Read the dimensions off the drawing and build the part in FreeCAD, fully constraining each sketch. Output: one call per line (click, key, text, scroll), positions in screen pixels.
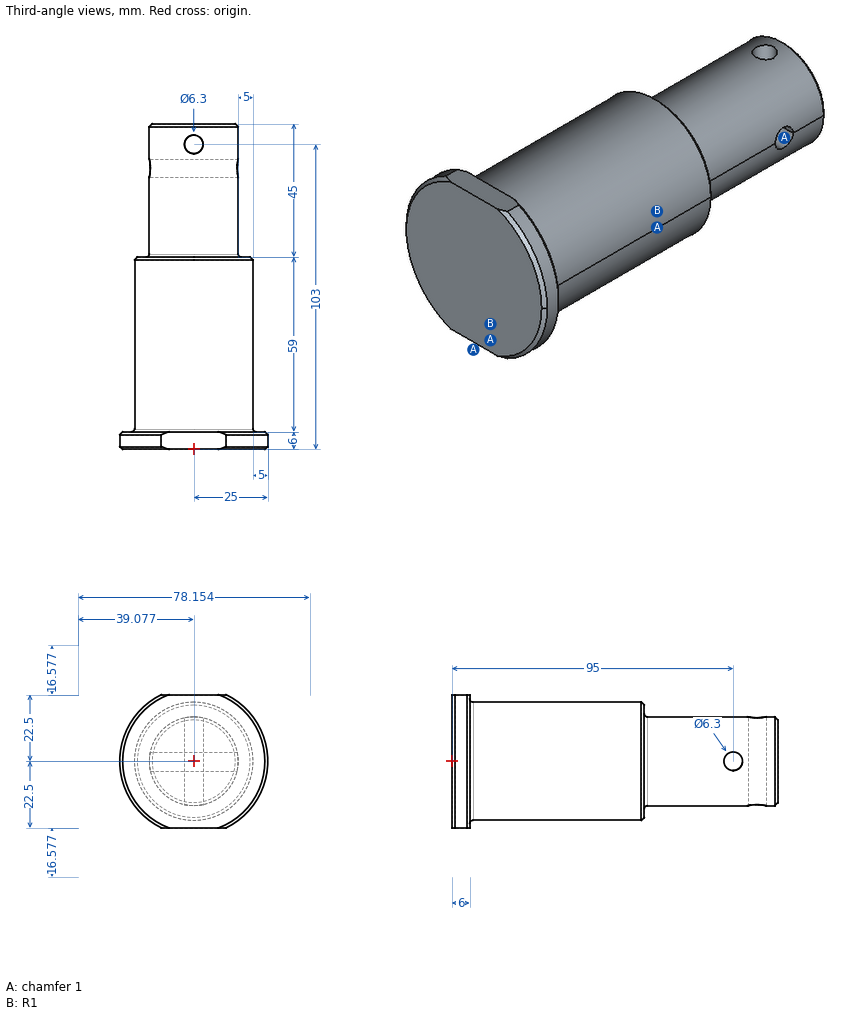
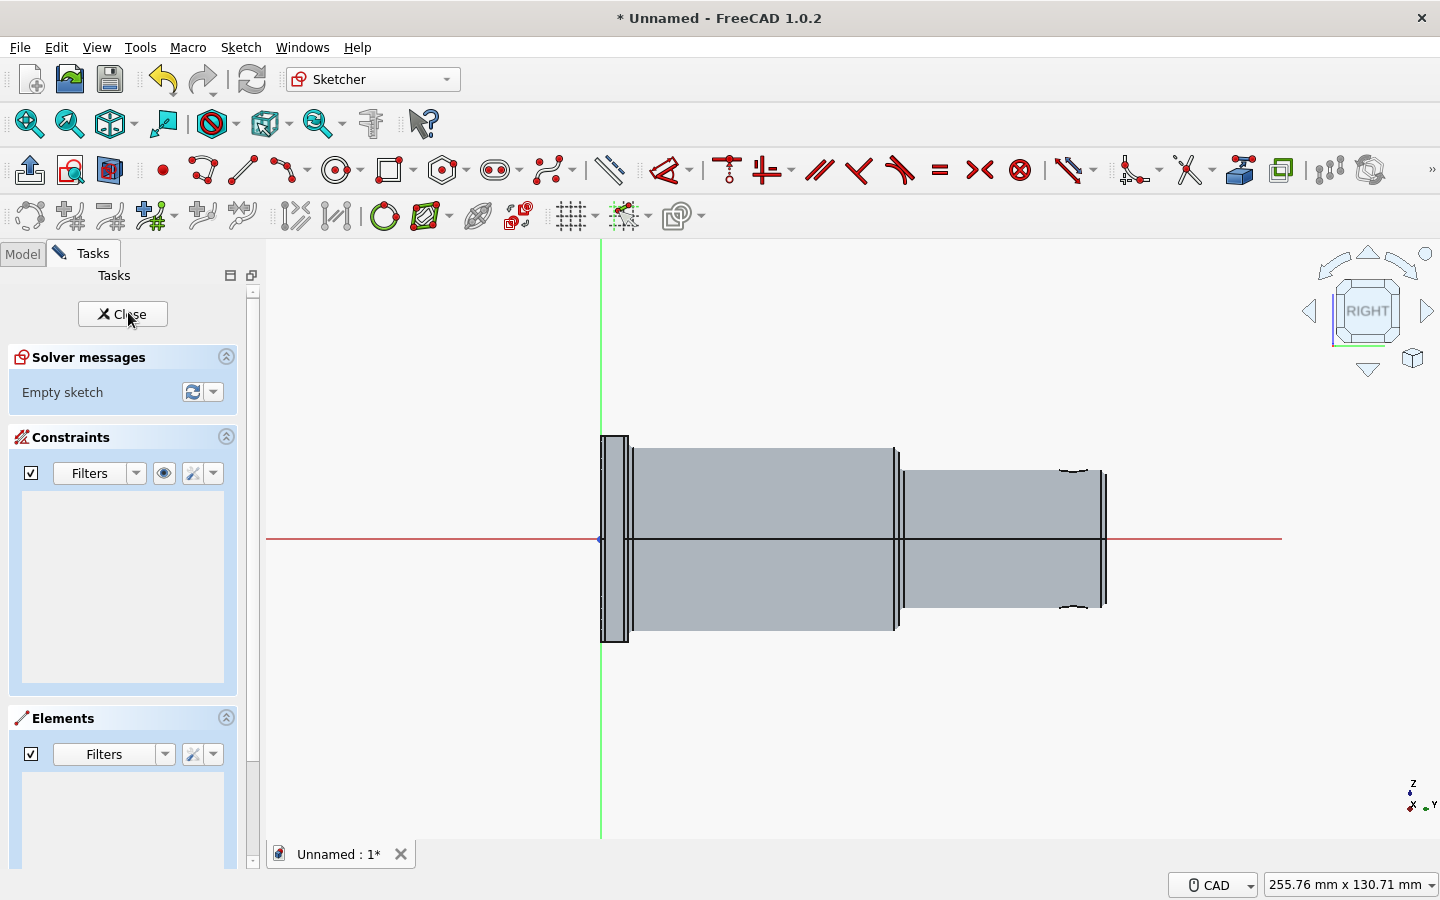
key(q)
key(s)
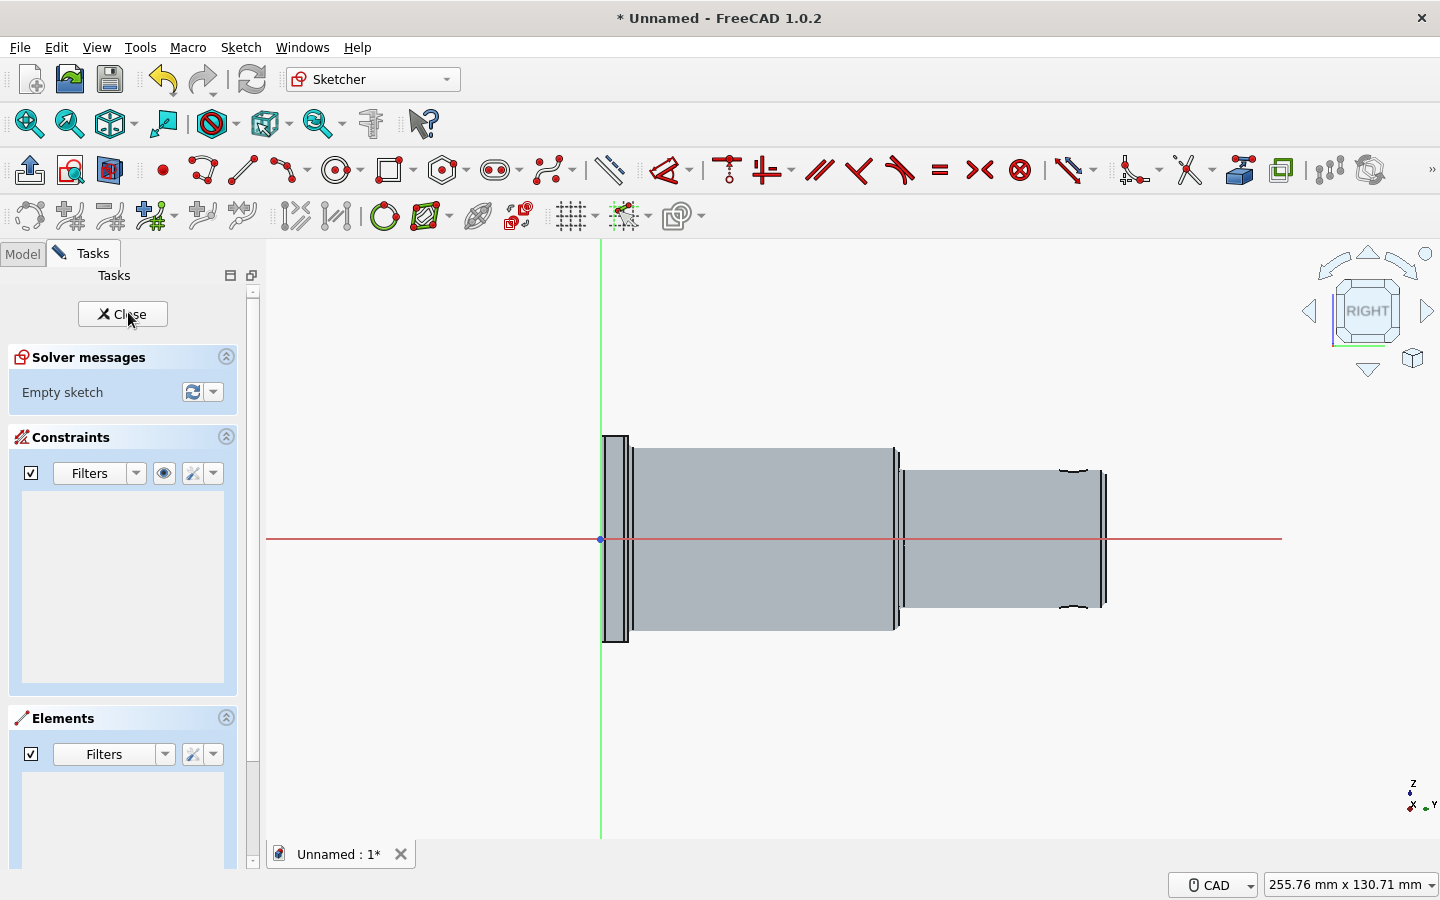
scroll(1057, 539, up, 13)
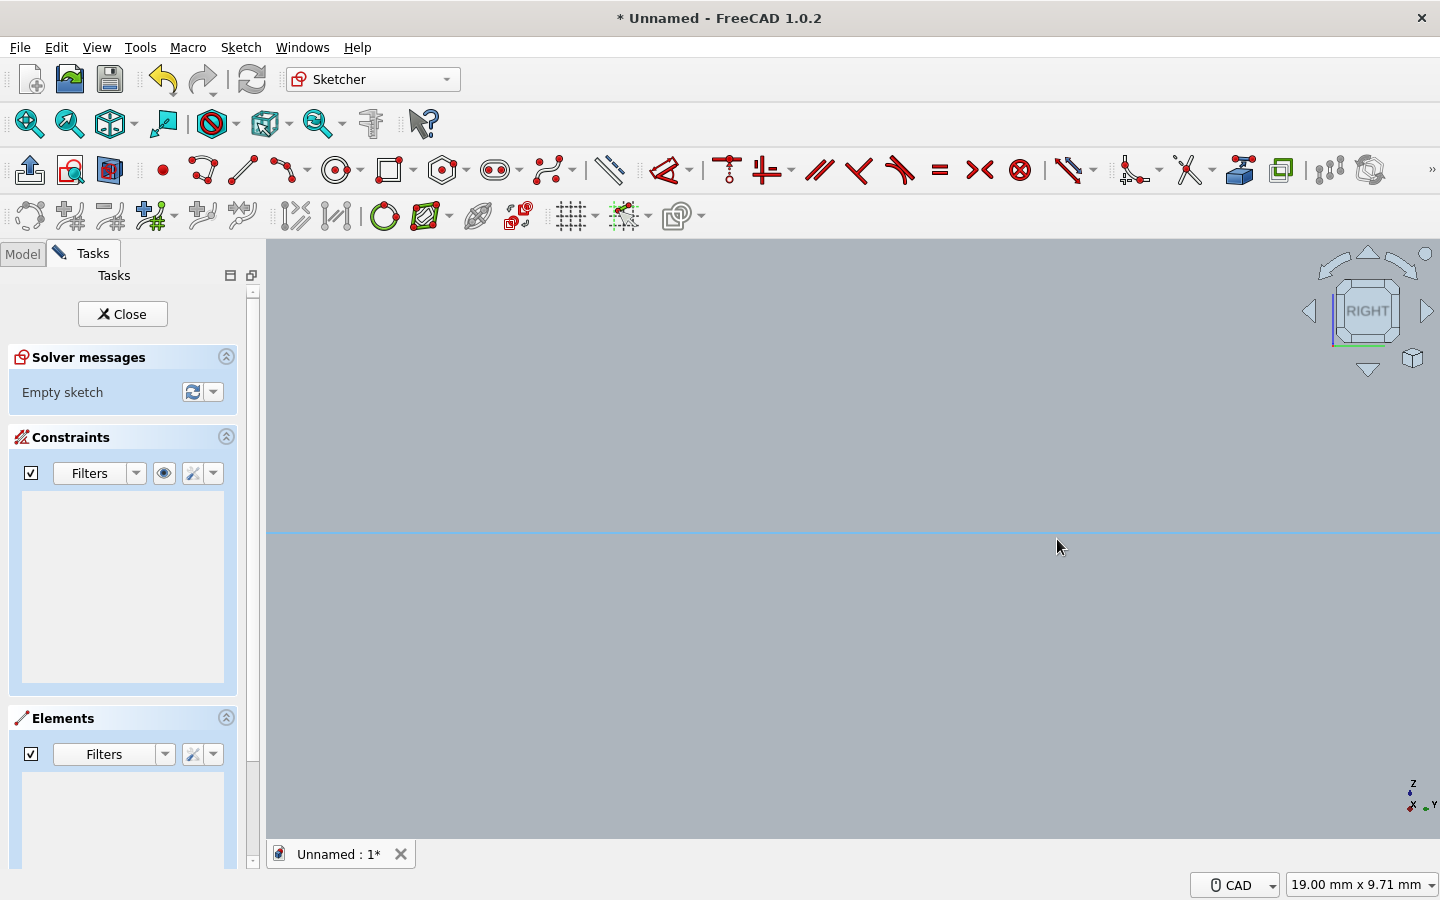
key(g)
key(c)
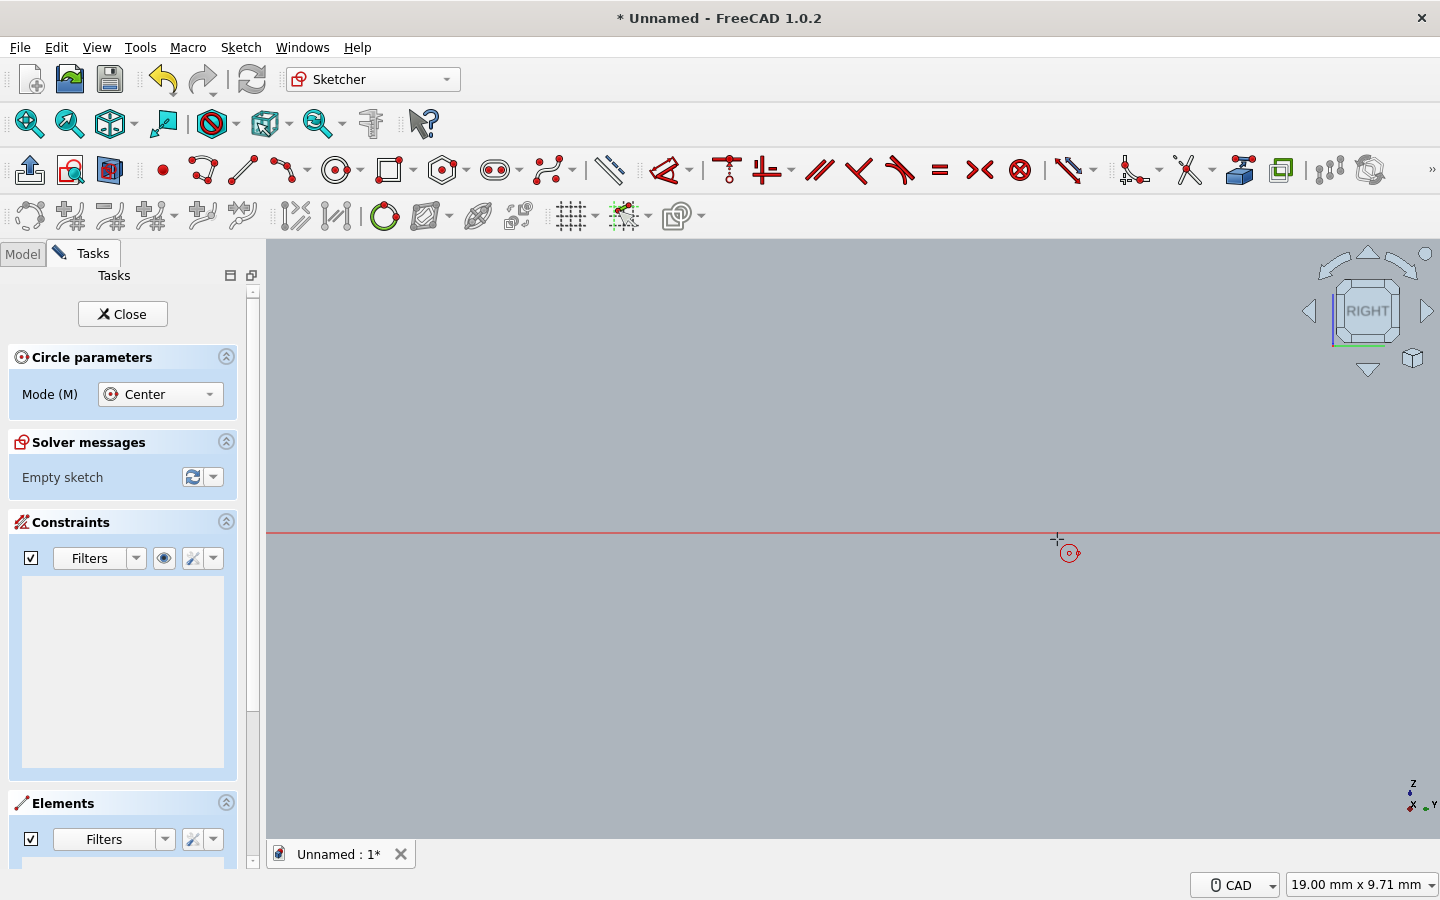
click(775, 533)
click(912, 396)
key(Escape)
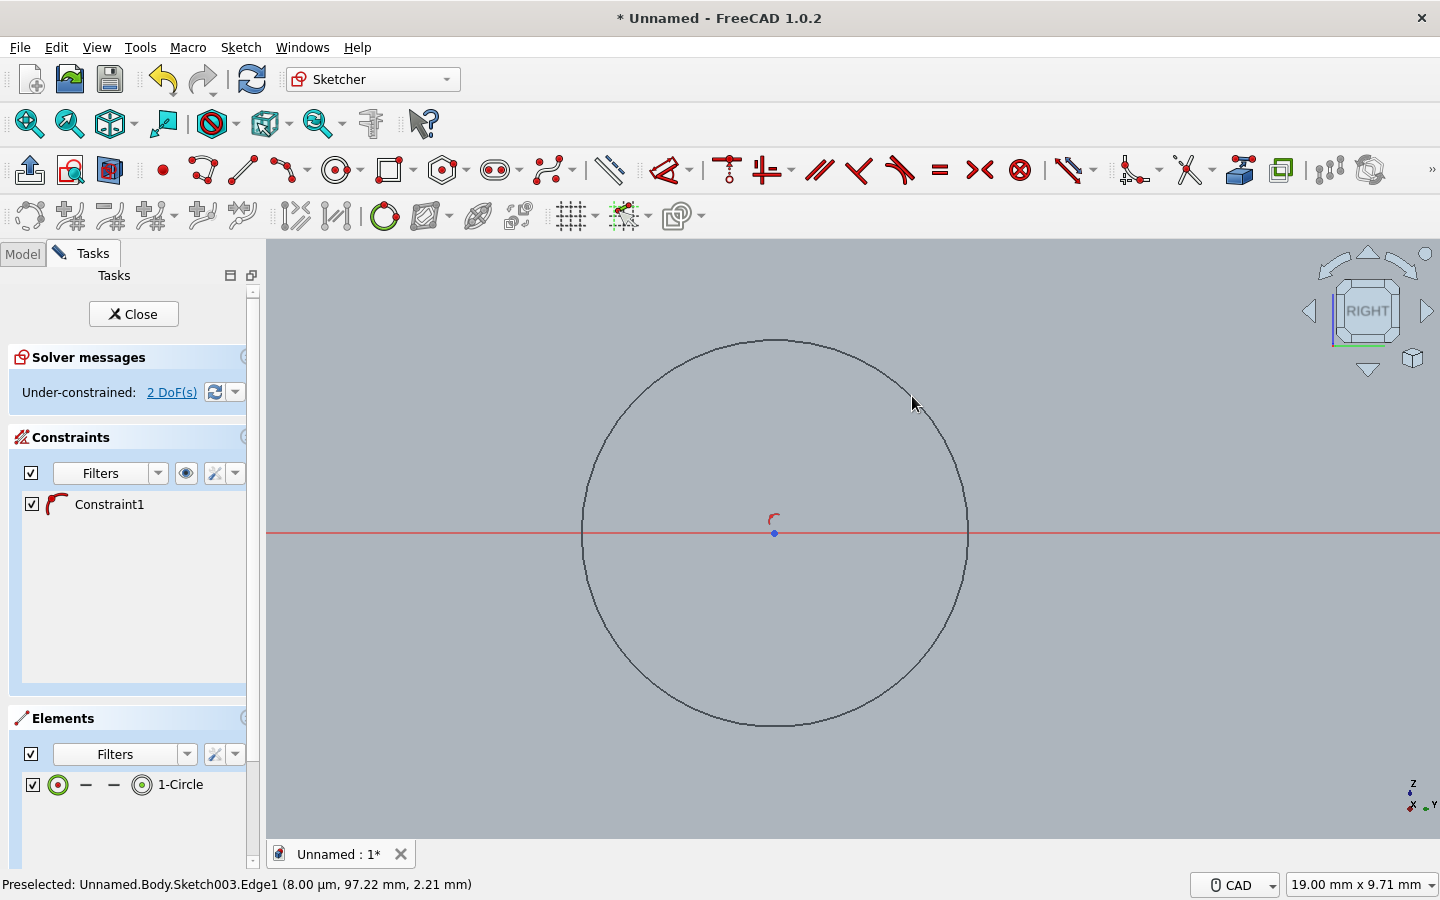
click(664, 170)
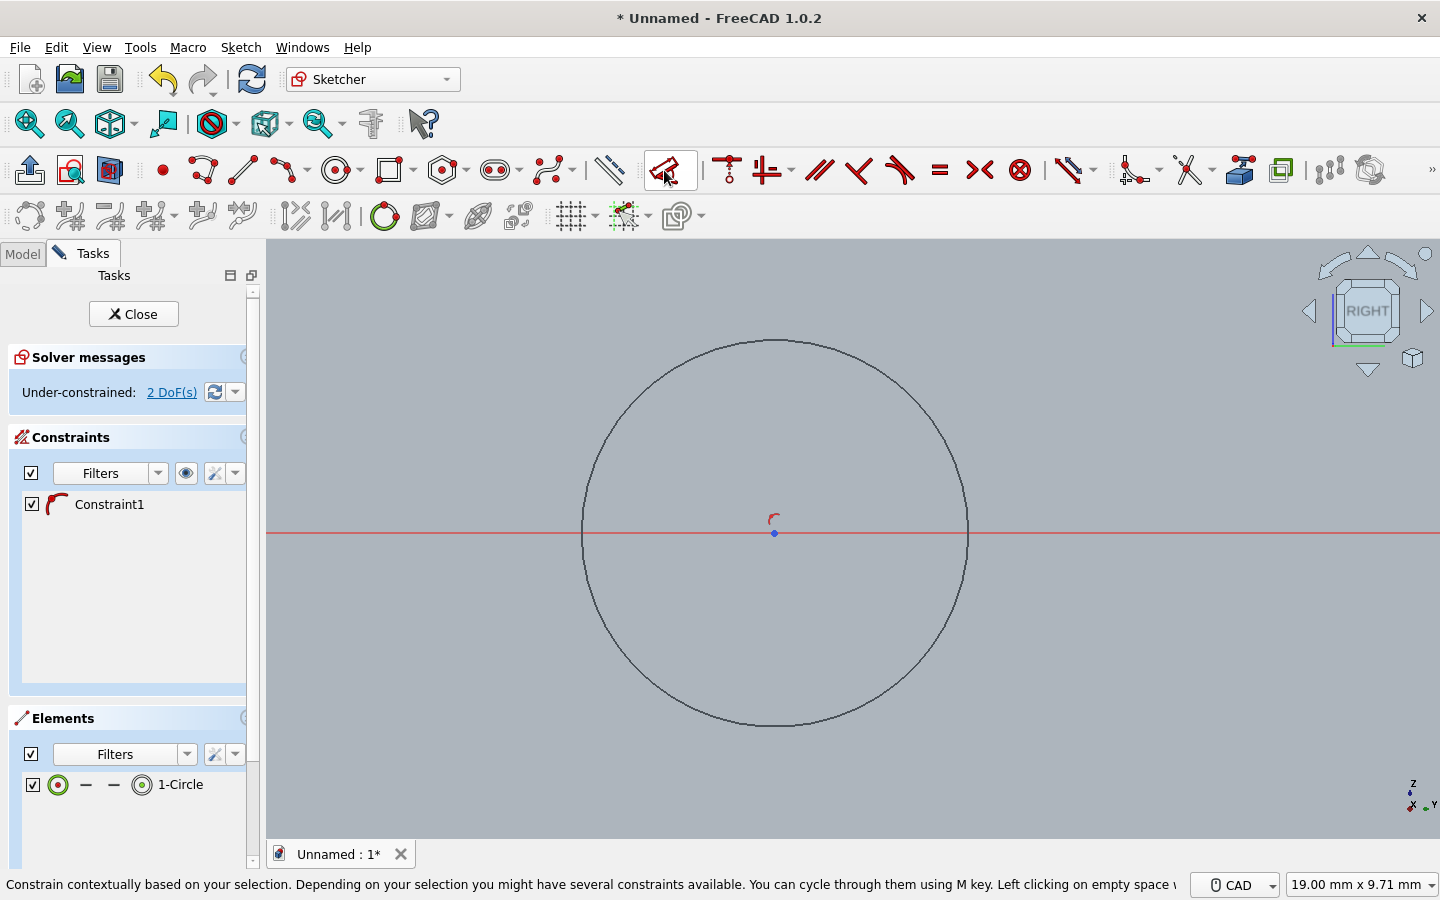
click(911, 396)
click(934, 373)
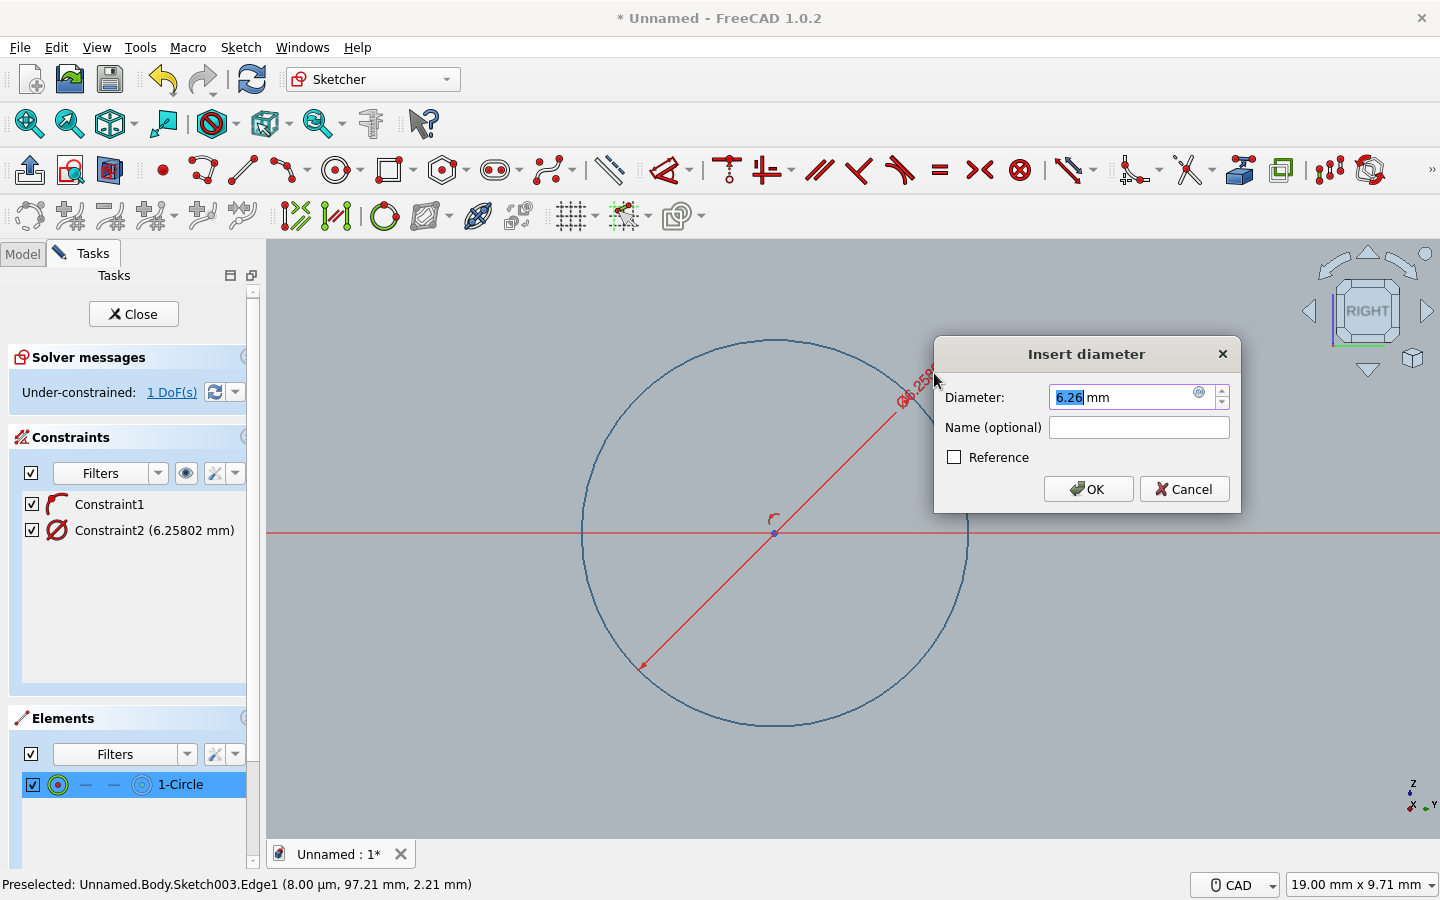
text(6.3)
key(Return)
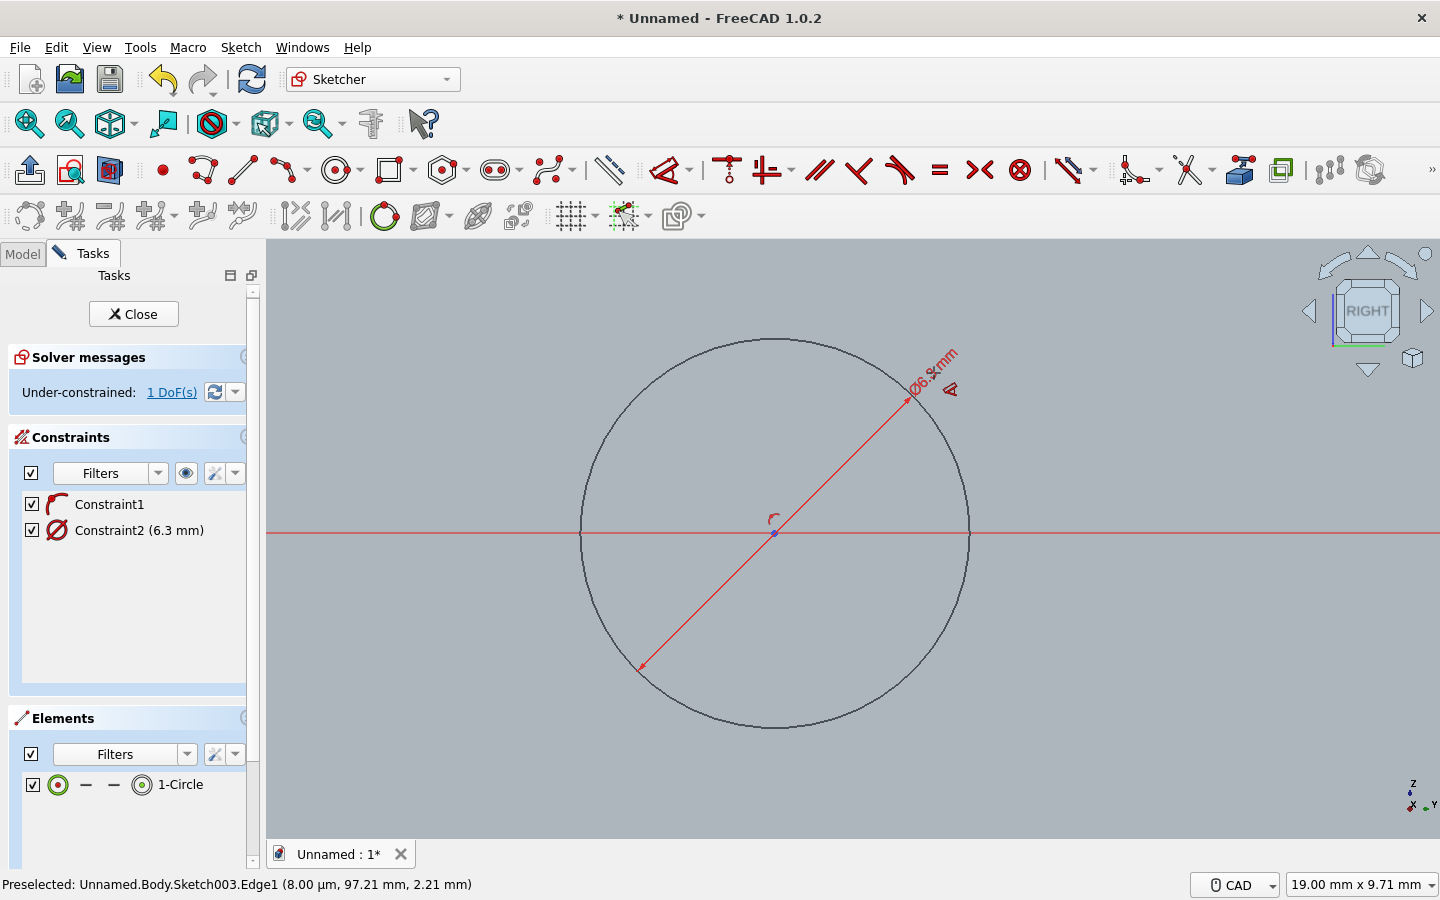
click(775, 533)
click(534, 567)